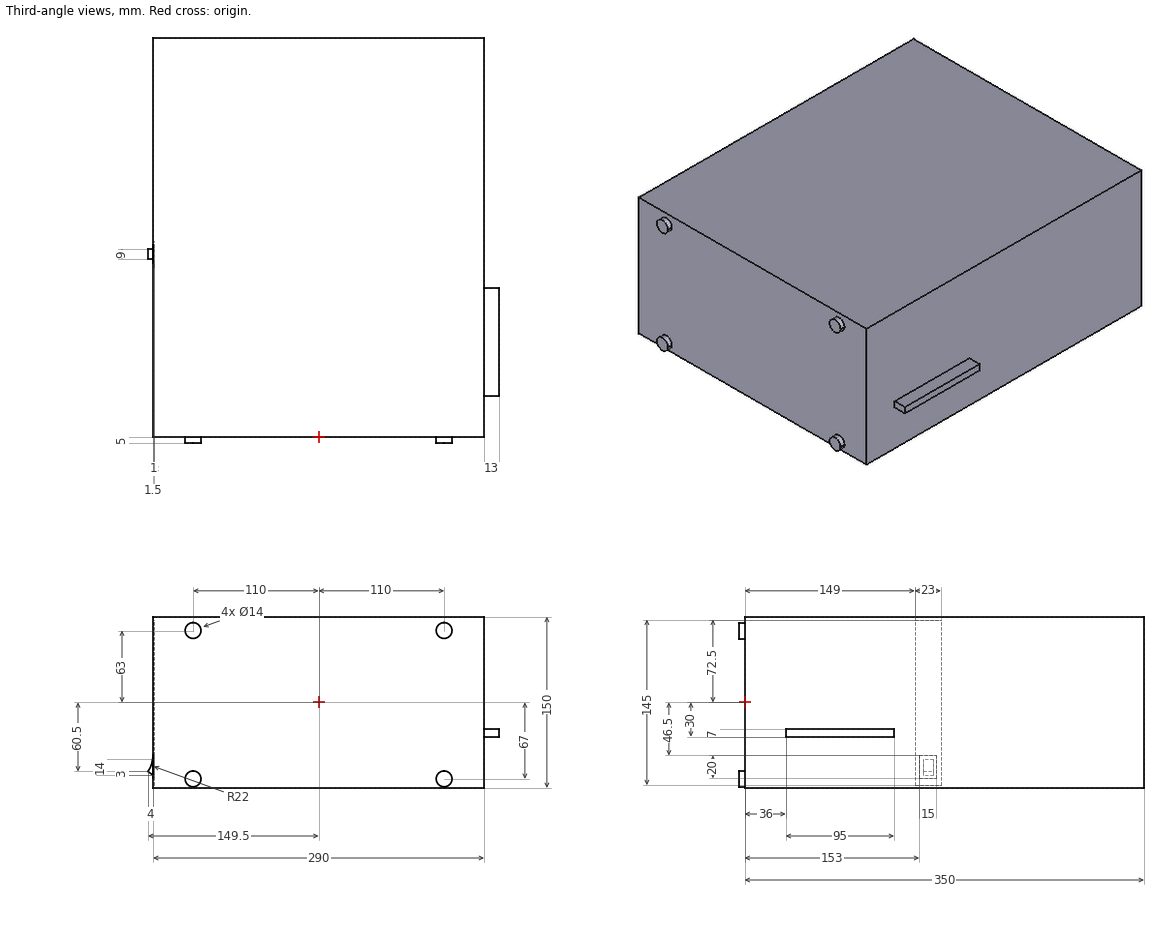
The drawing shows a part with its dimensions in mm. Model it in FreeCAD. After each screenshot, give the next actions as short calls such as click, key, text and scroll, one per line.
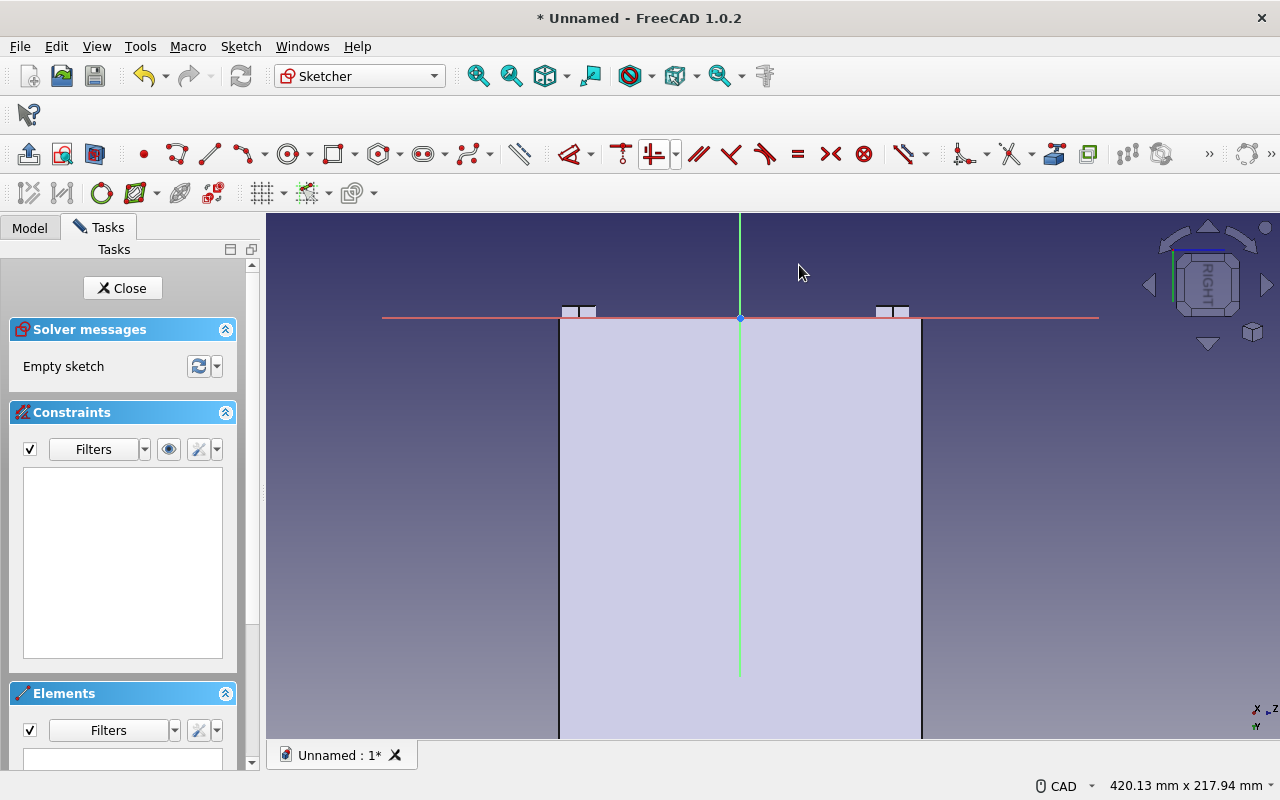
click(332, 154)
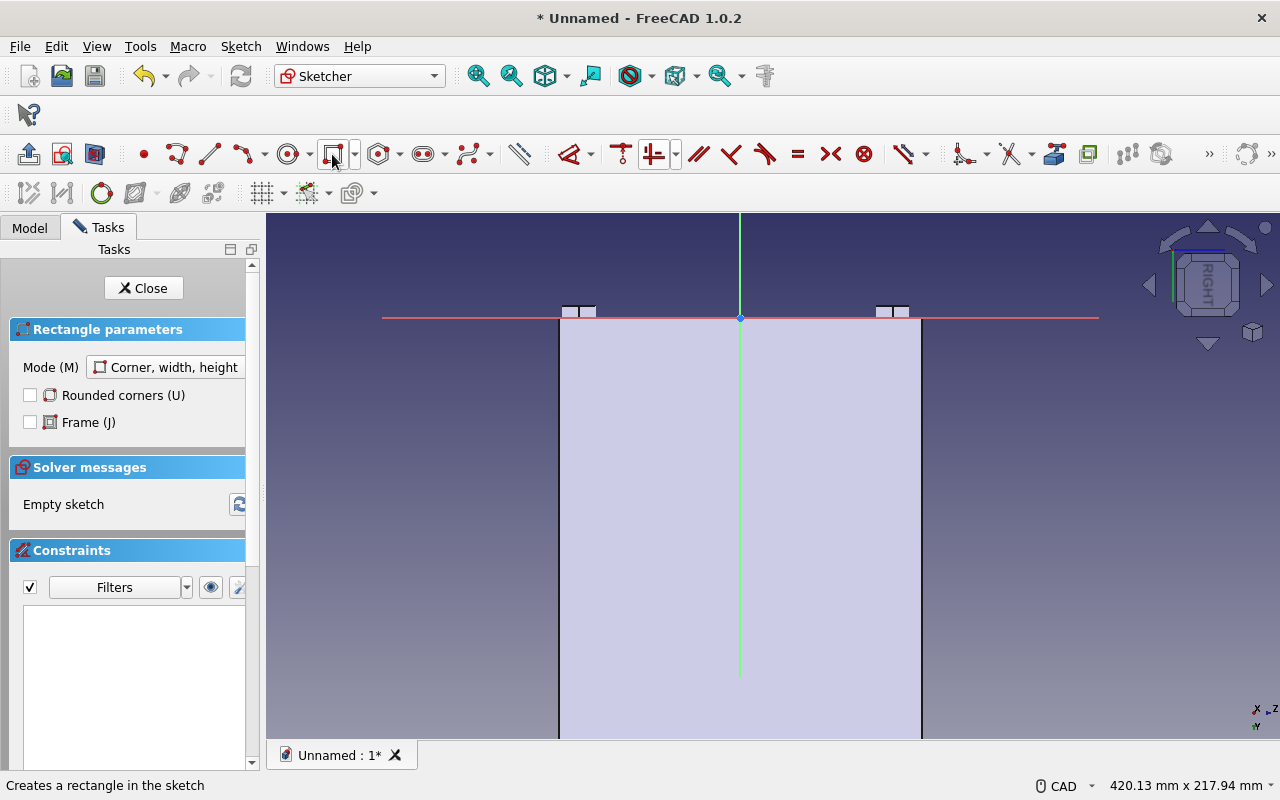
click(668, 405)
click(685, 634)
key(Escape)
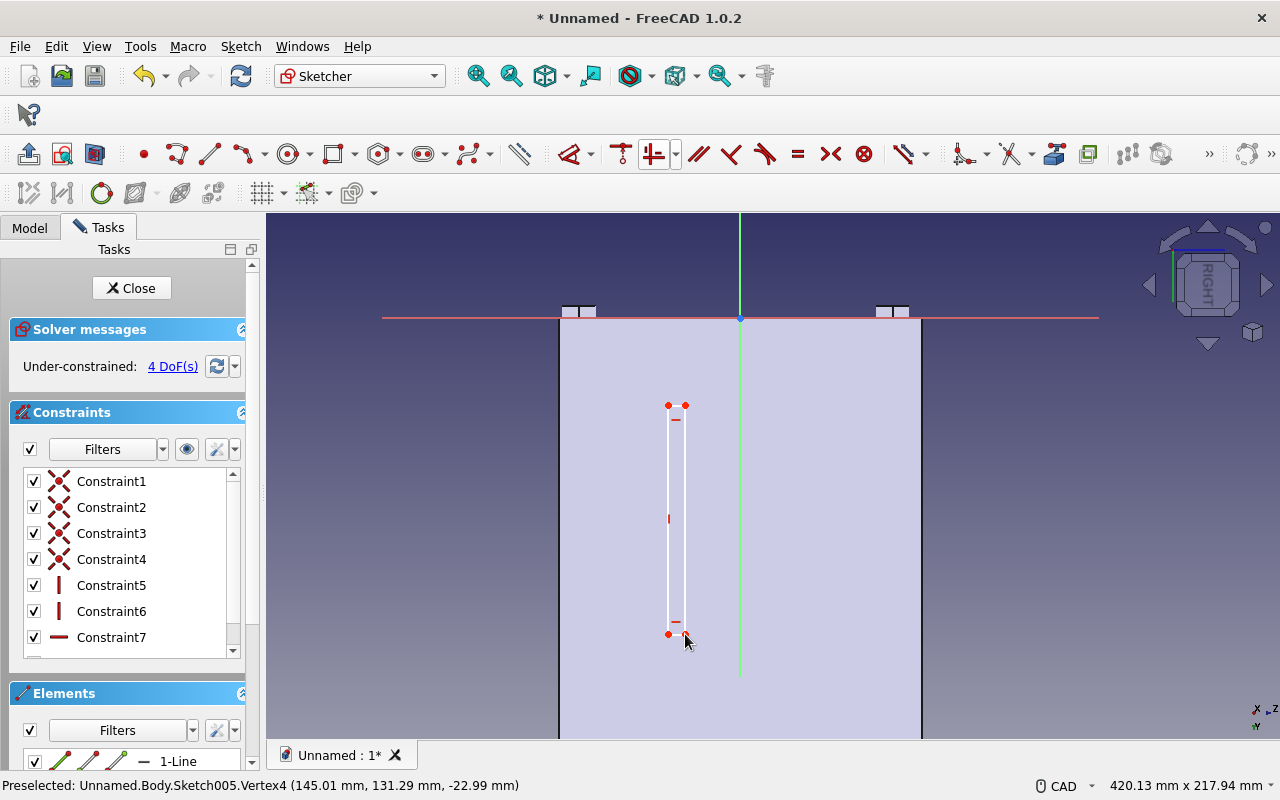
click(568, 154)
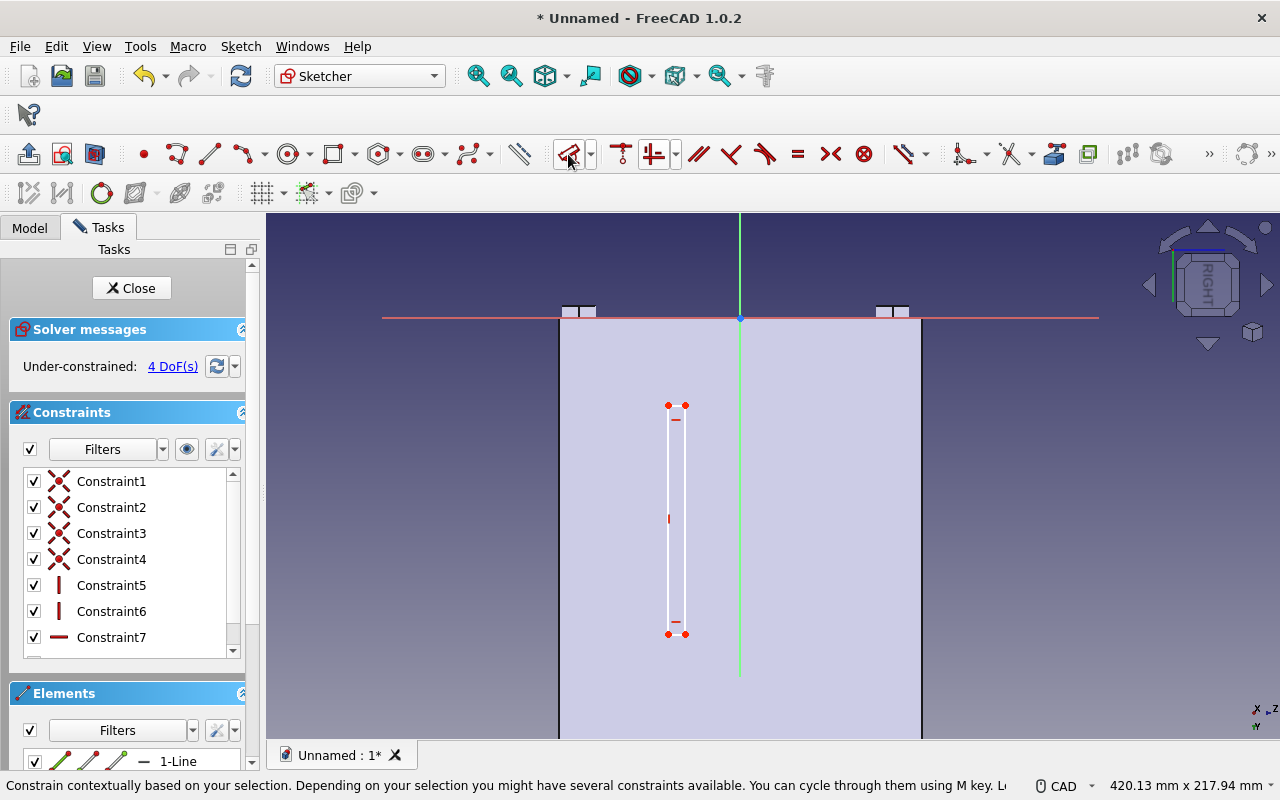
scroll(676, 635, up, 5)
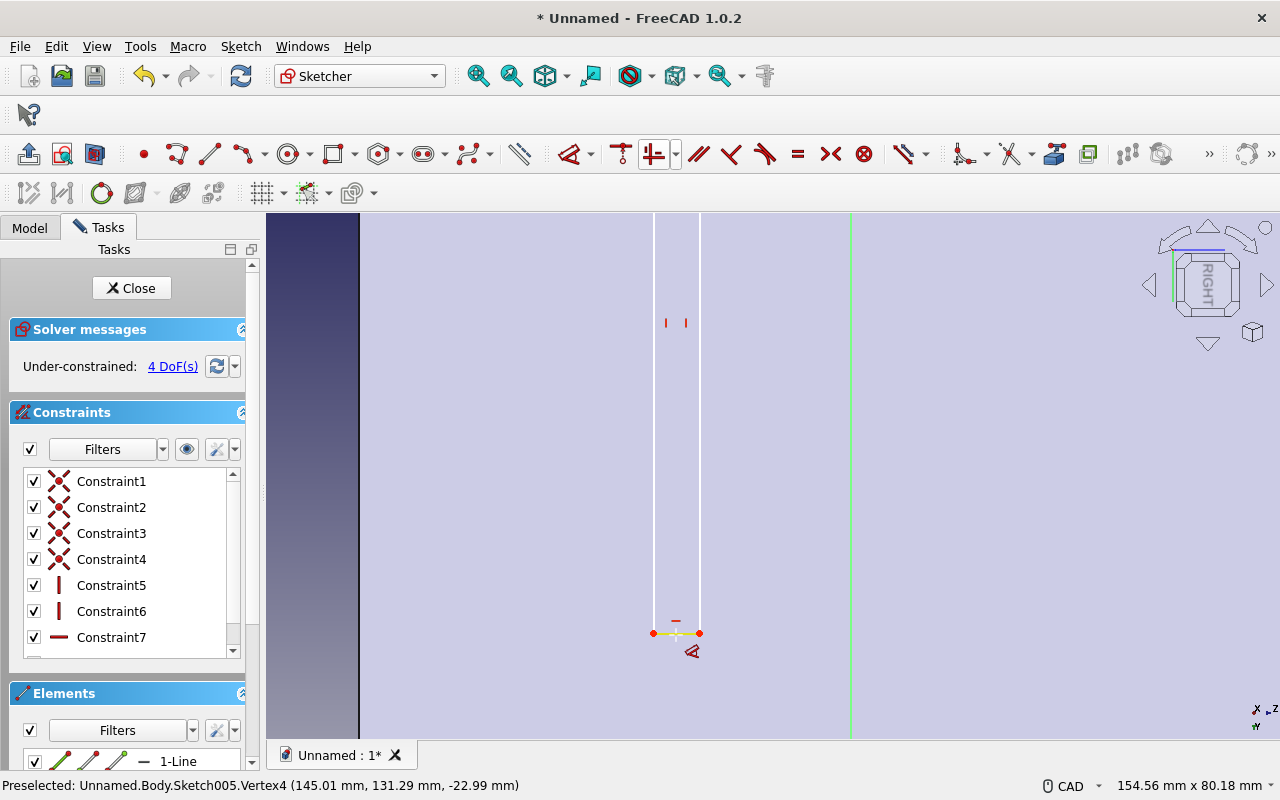
click(677, 634)
click(677, 668)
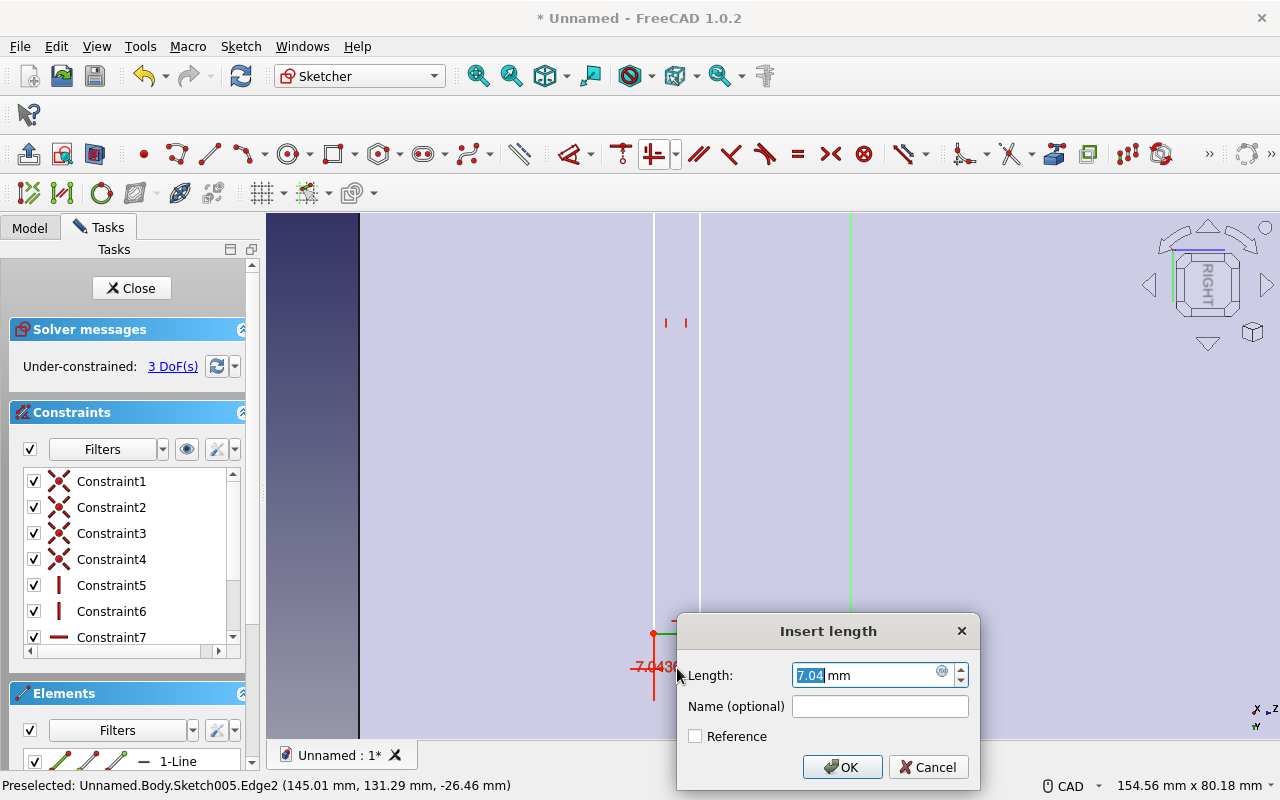
text(7)
key(Return)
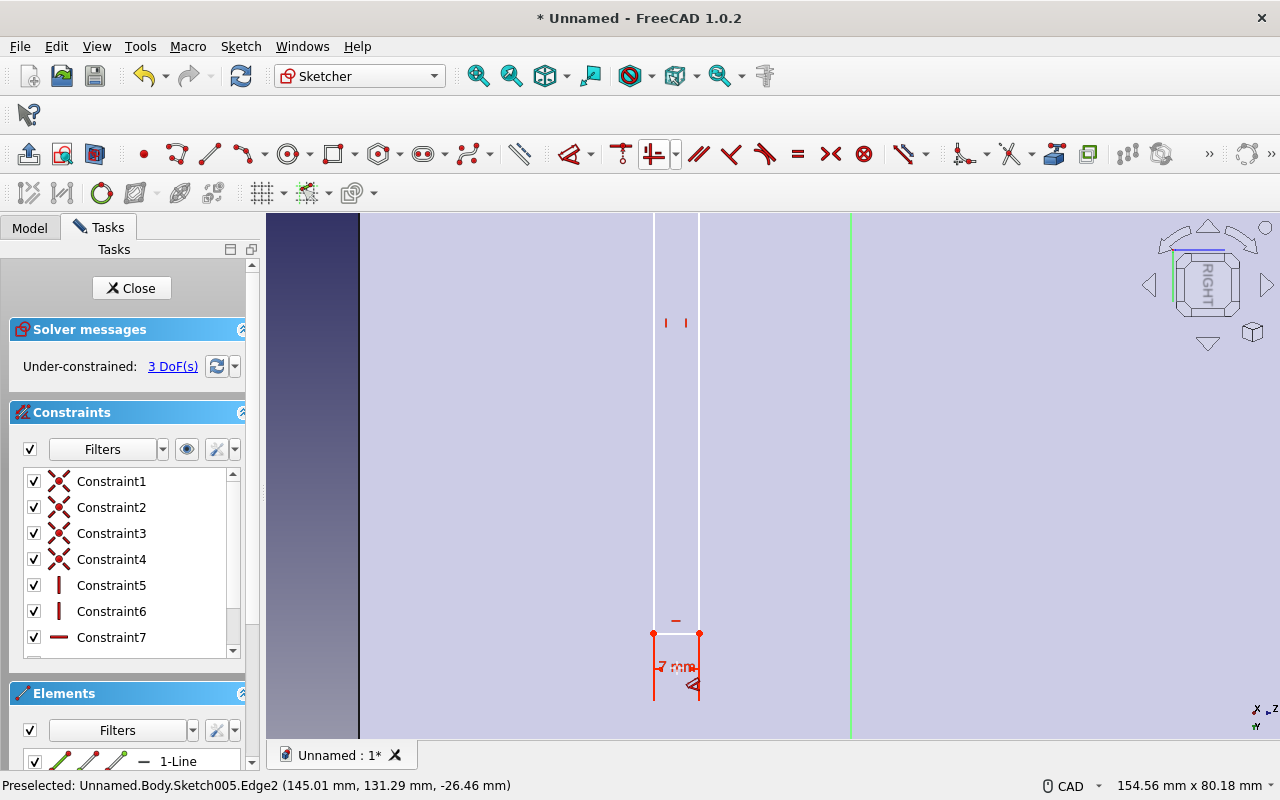
click(654, 447)
click(620, 437)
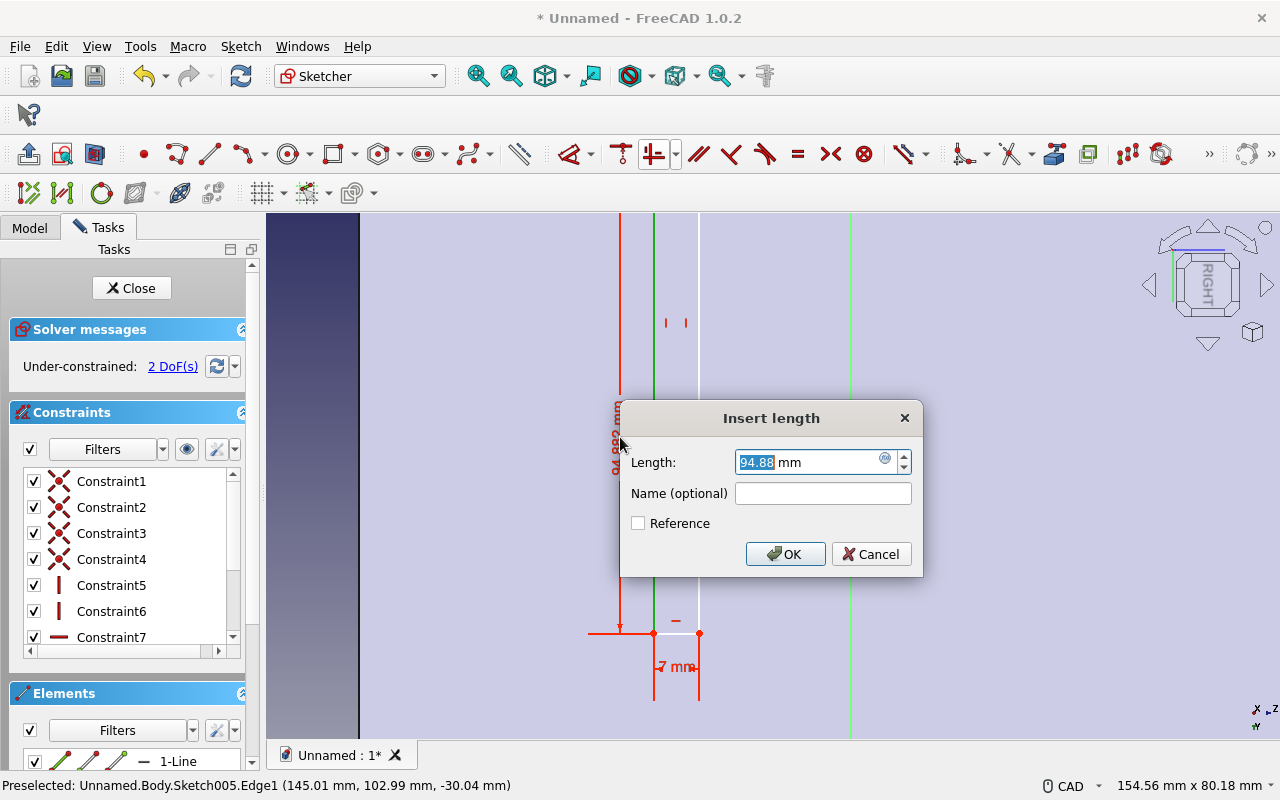
text(95)
key(Return)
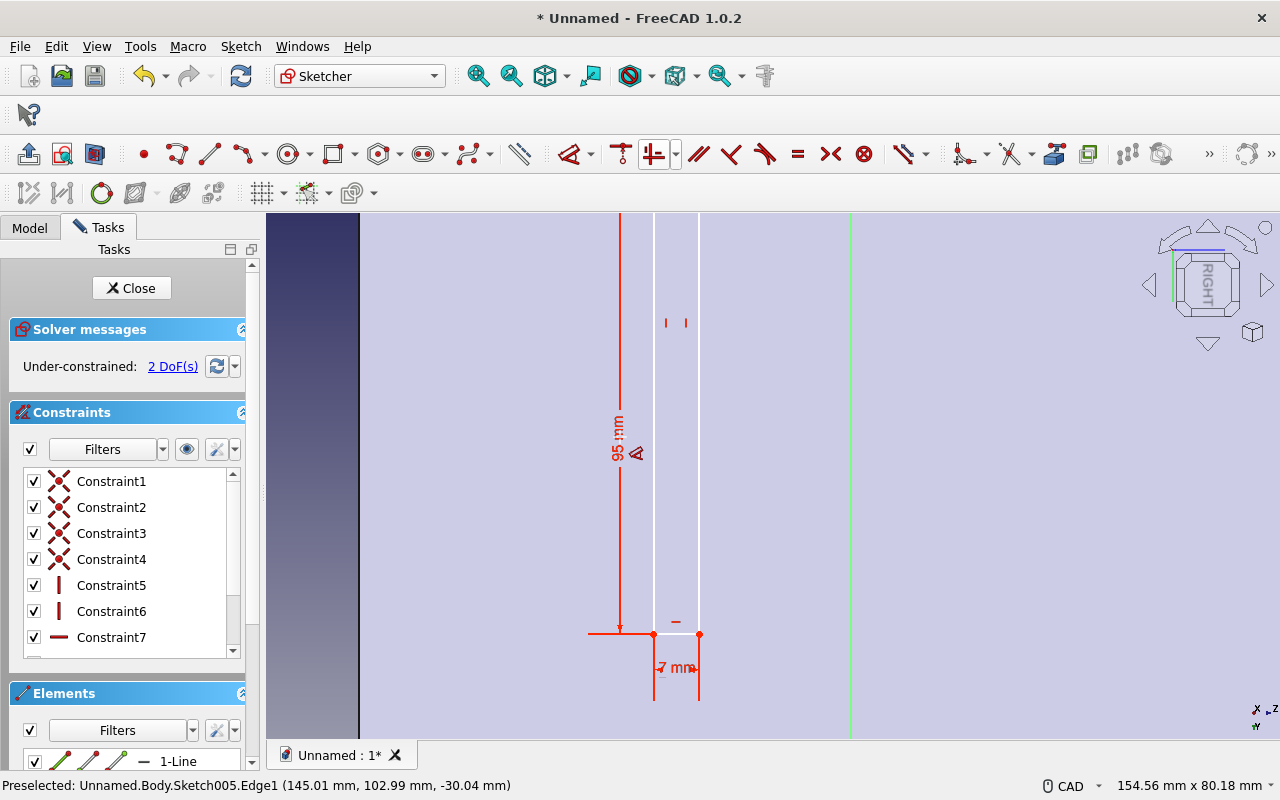
scroll(677, 635, down, 5)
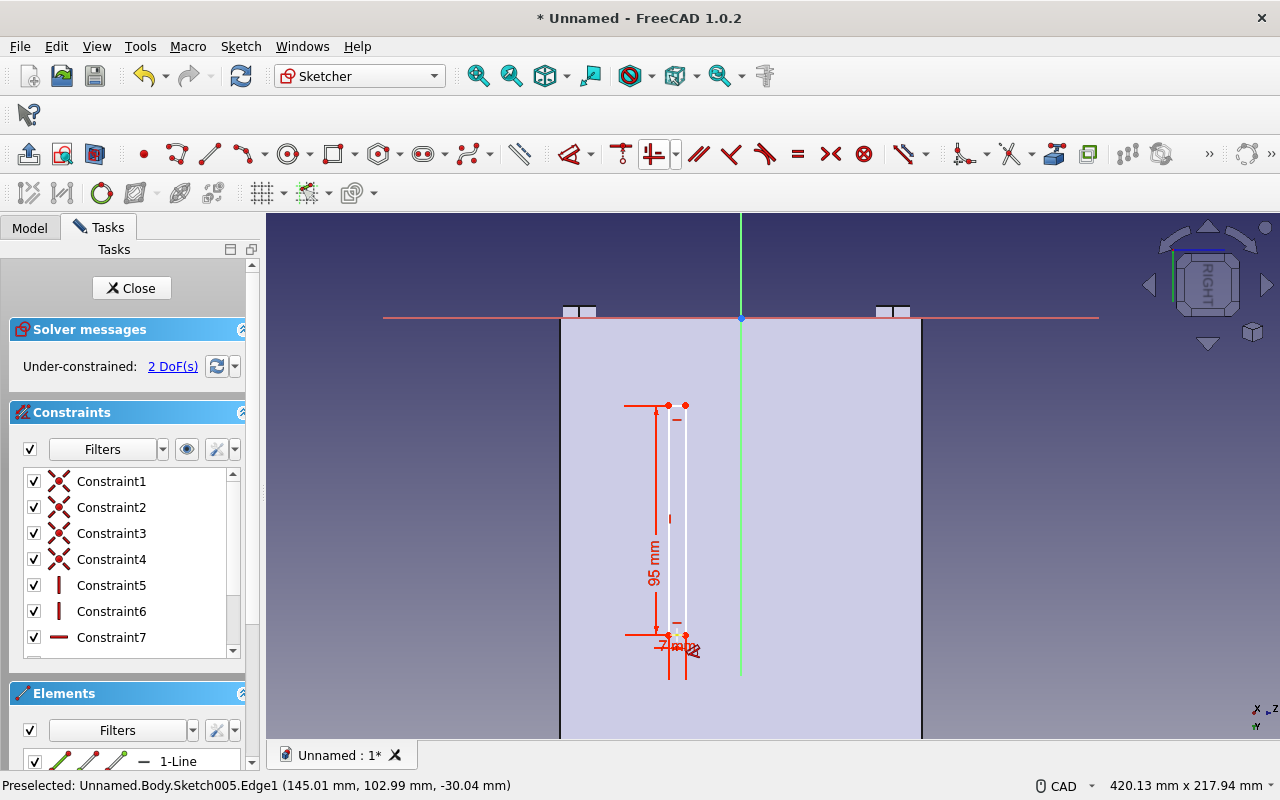
click(669, 406)
click(705, 284)